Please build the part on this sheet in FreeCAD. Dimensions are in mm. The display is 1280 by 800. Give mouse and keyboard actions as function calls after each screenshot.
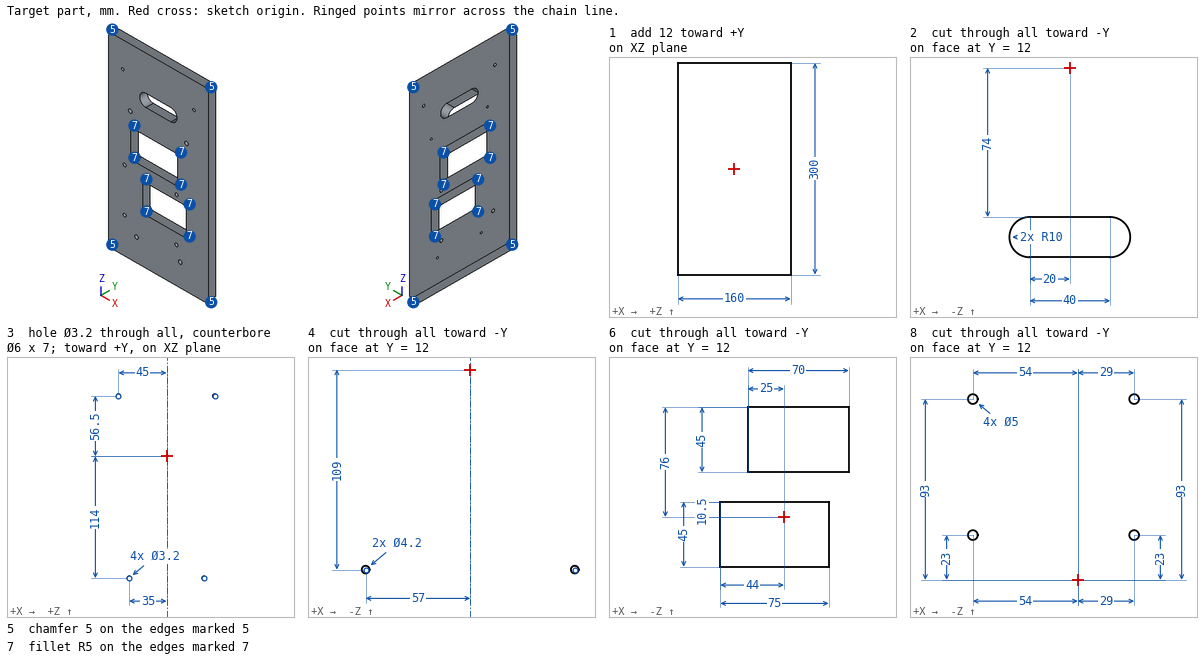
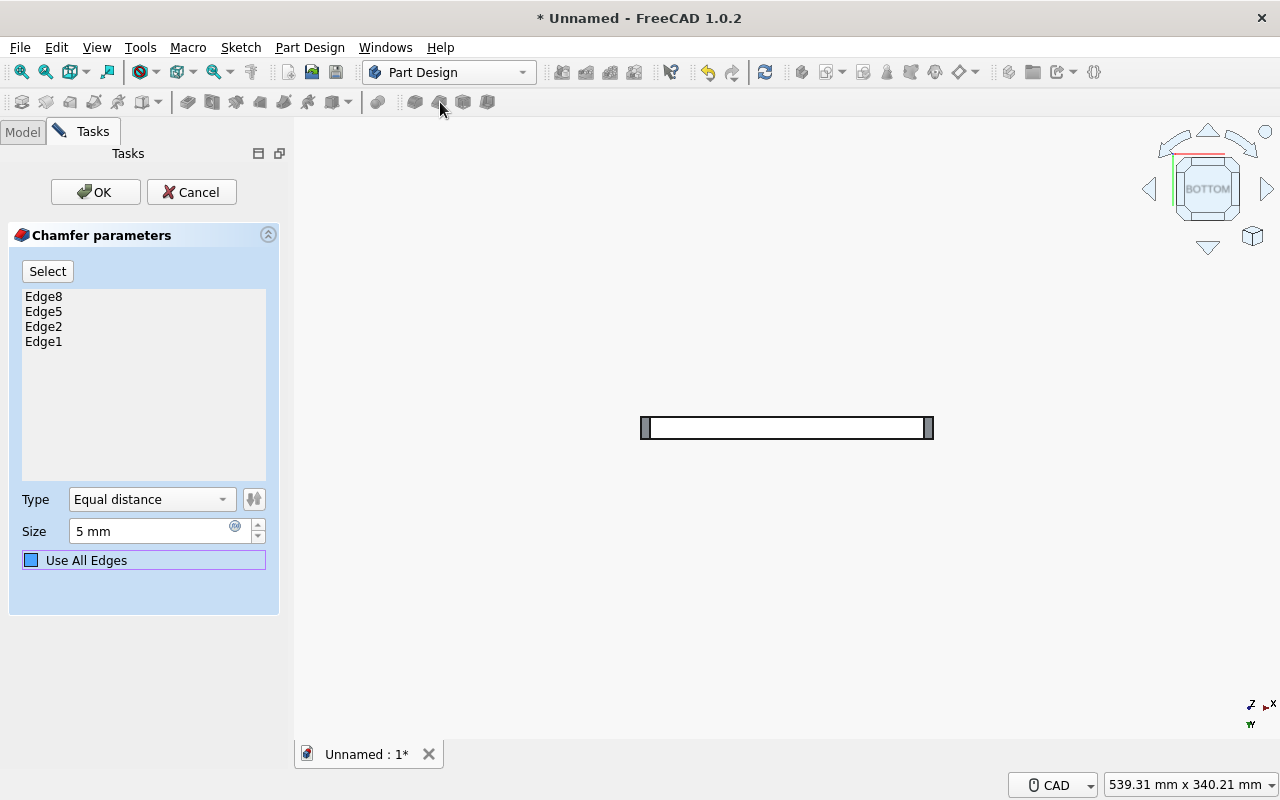
click(96, 192)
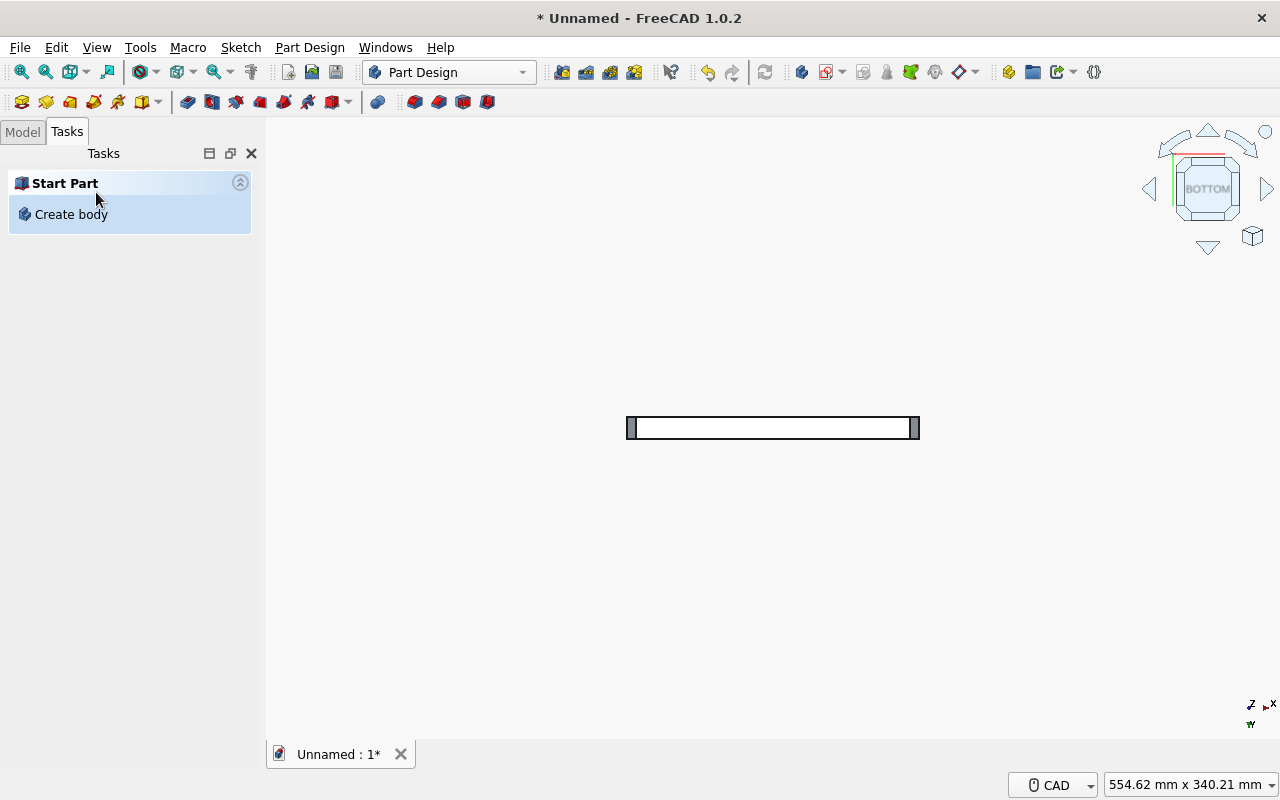
click(22, 72)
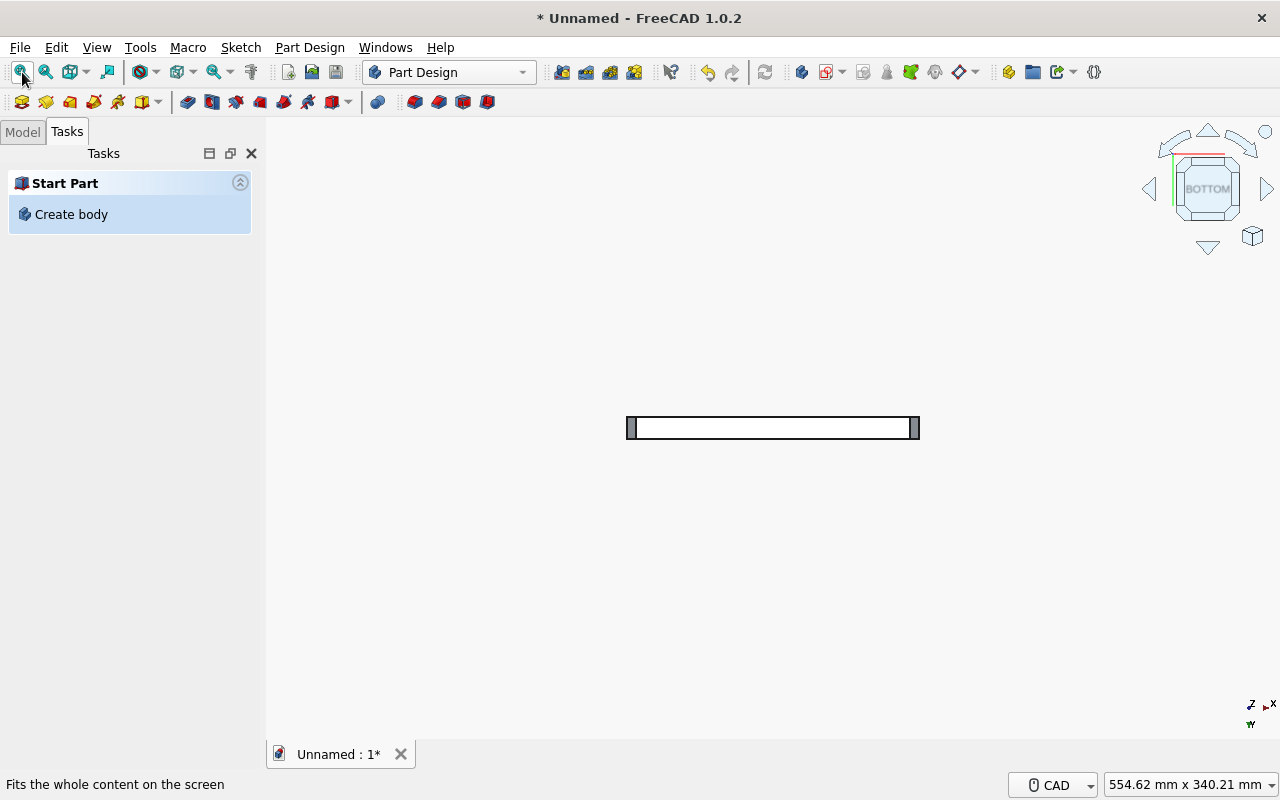
key(4)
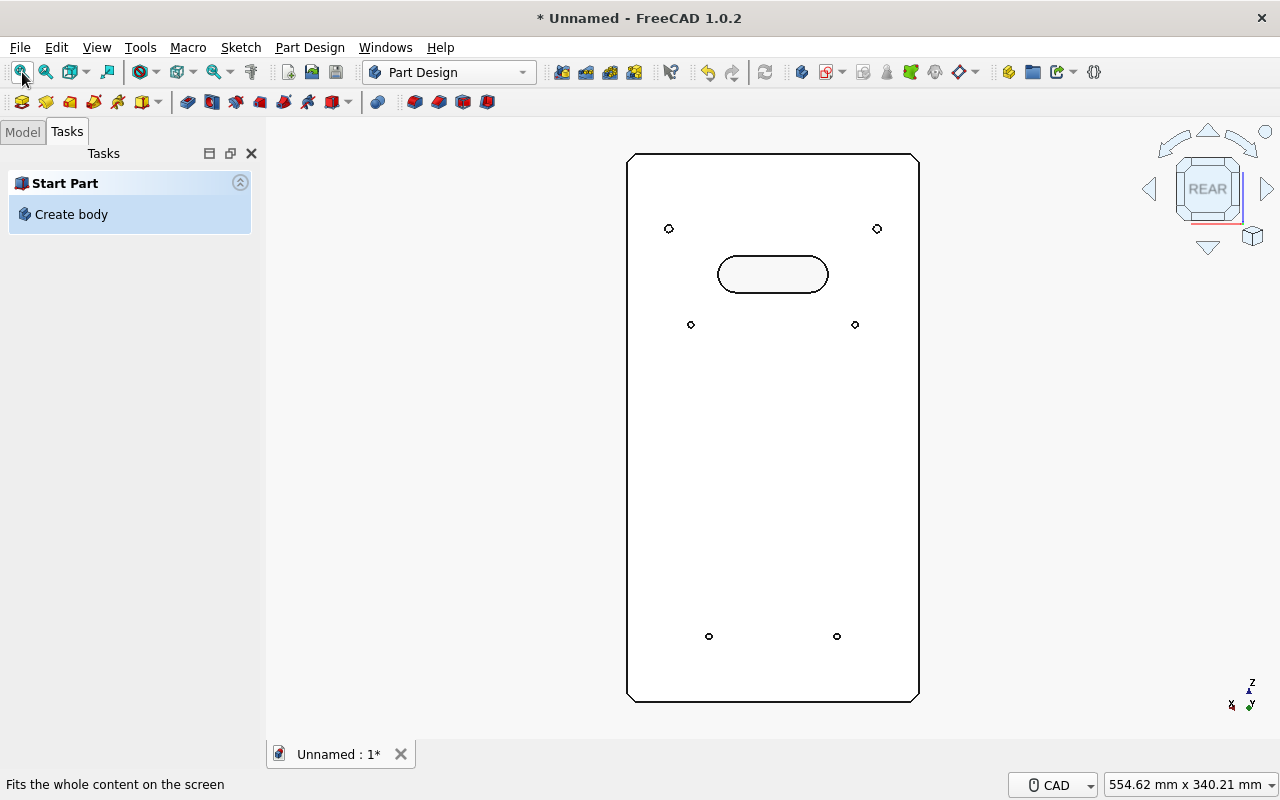
click(773, 505)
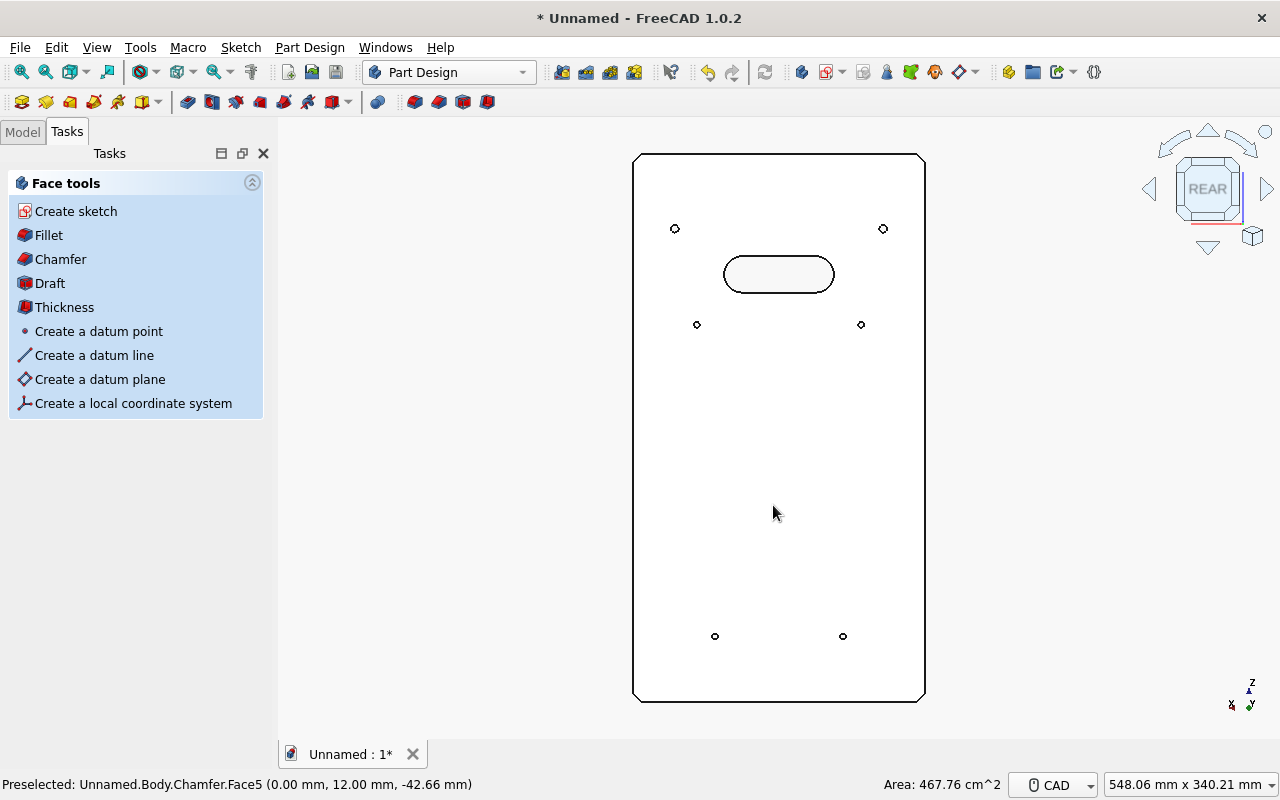
click(826, 72)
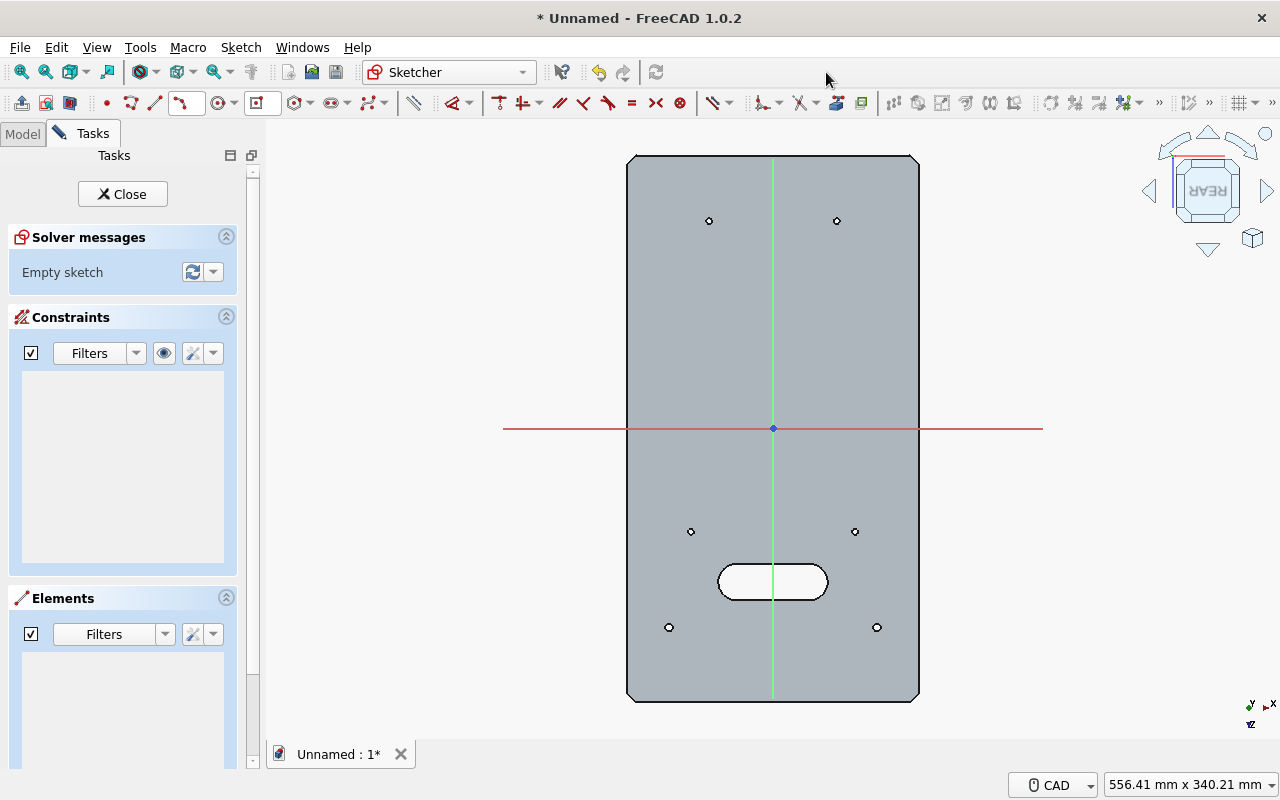
scroll(858, 345, up, 3)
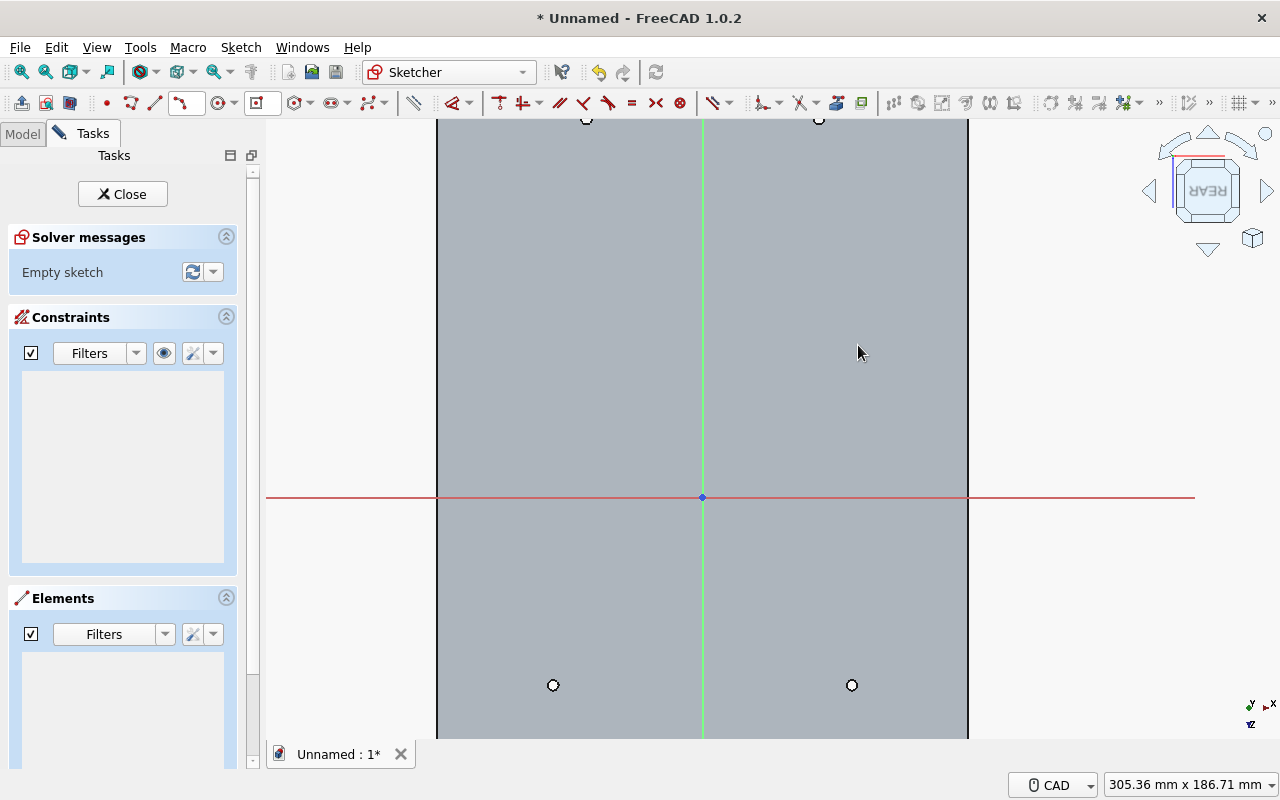
click(276, 104)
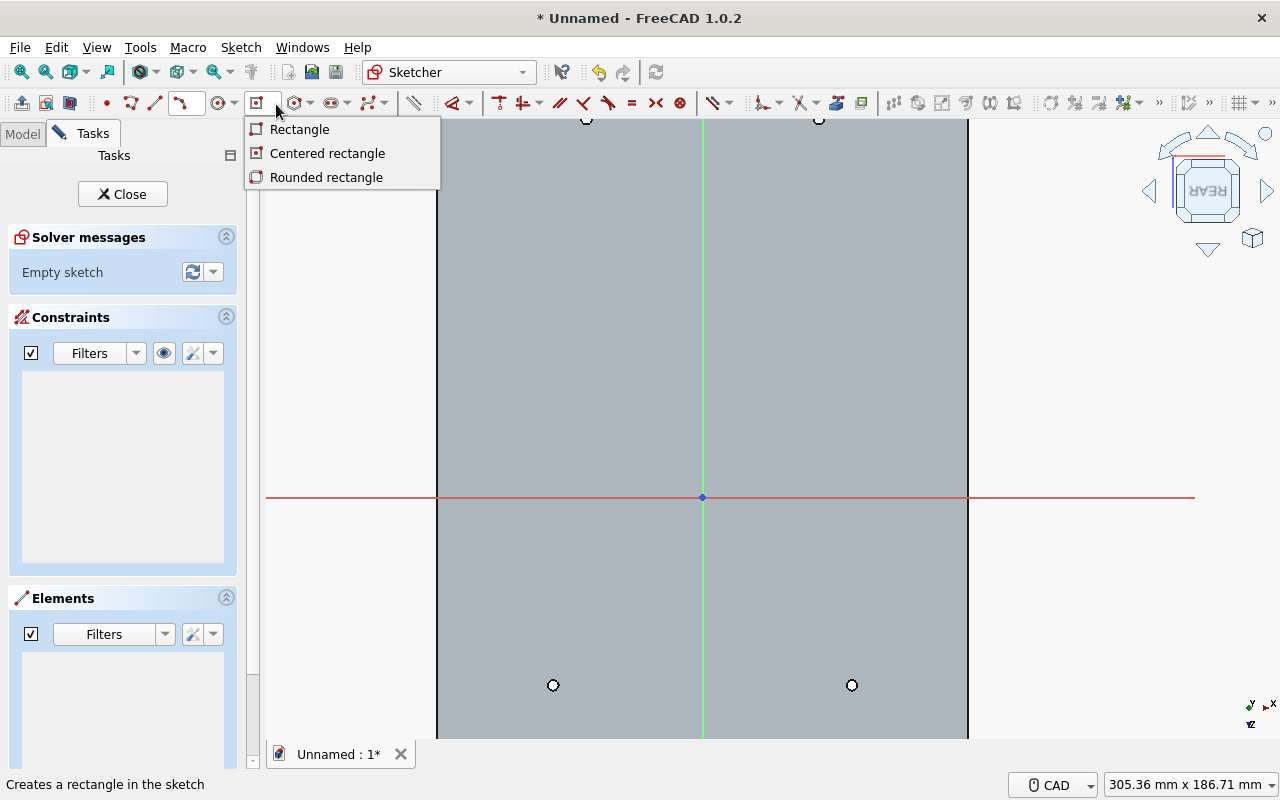
click(342, 129)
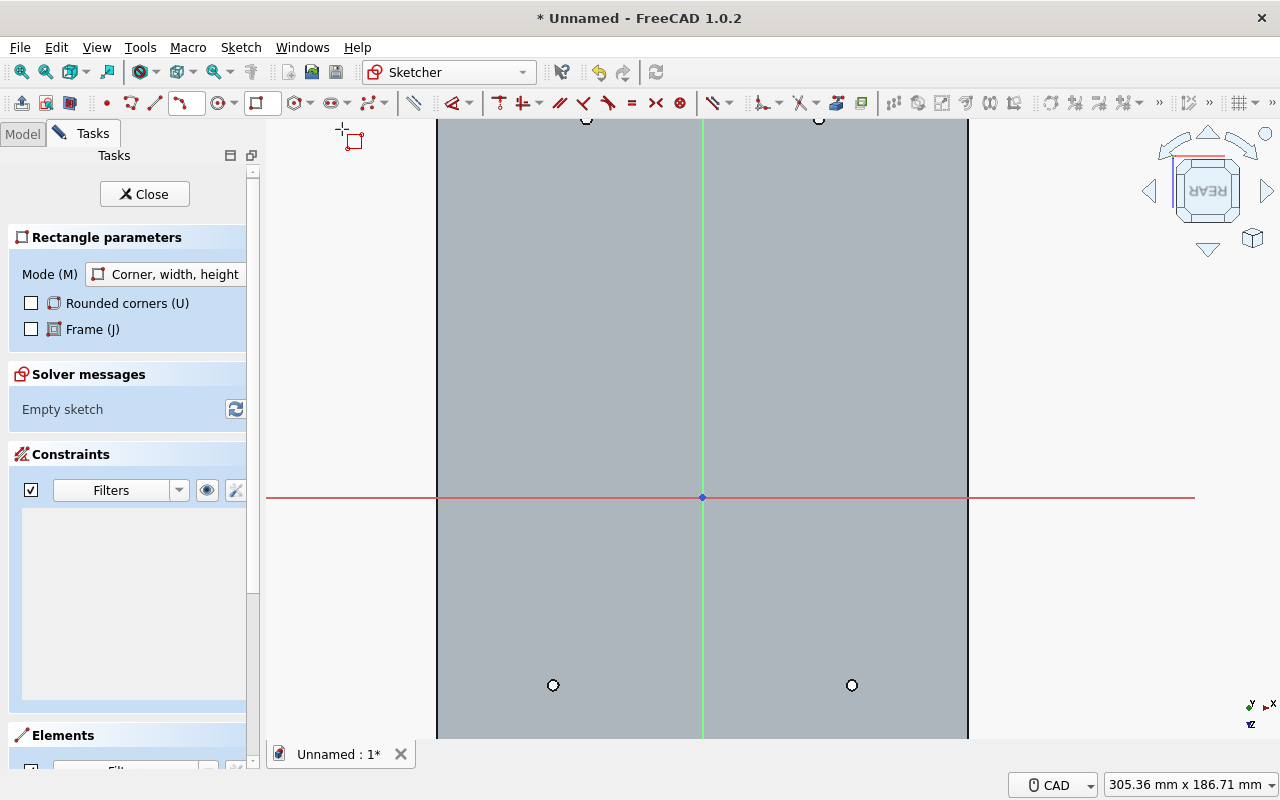
click(620, 245)
click(852, 395)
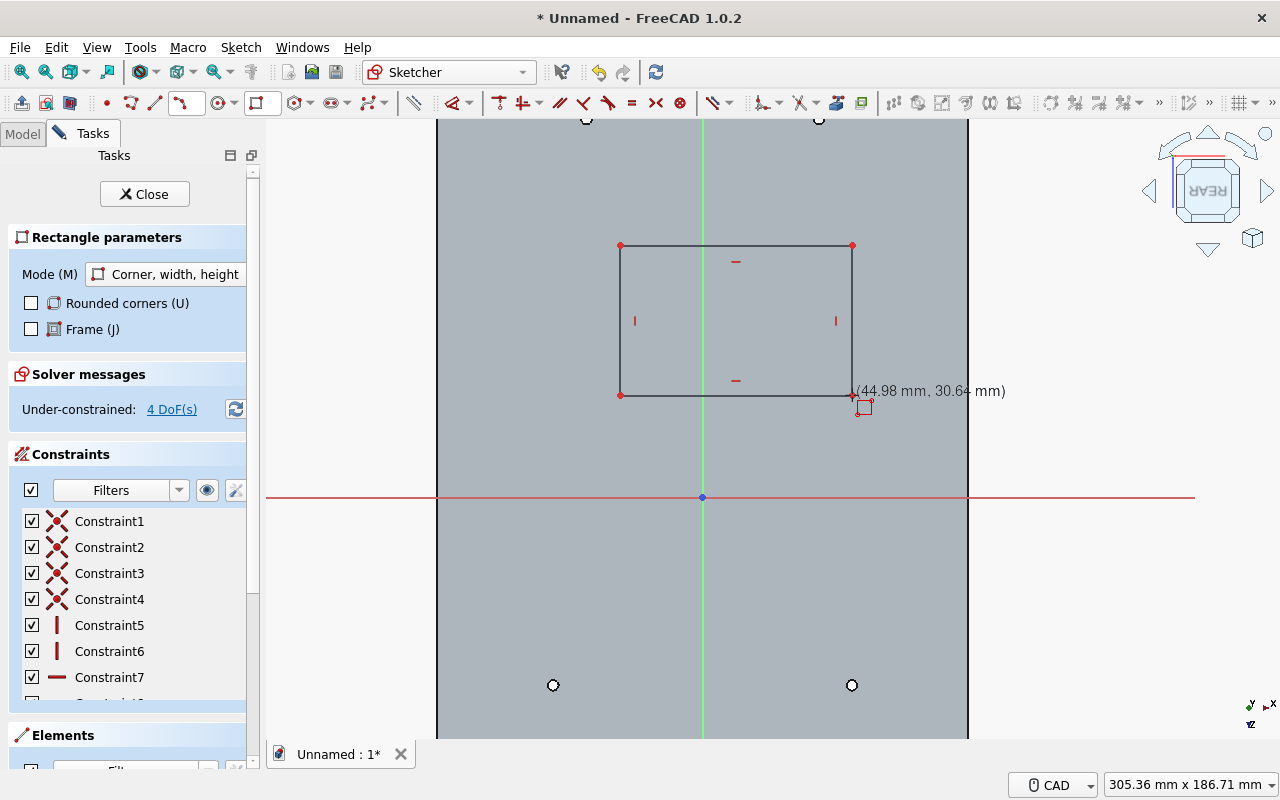
click(557, 463)
click(806, 612)
key(Escape)